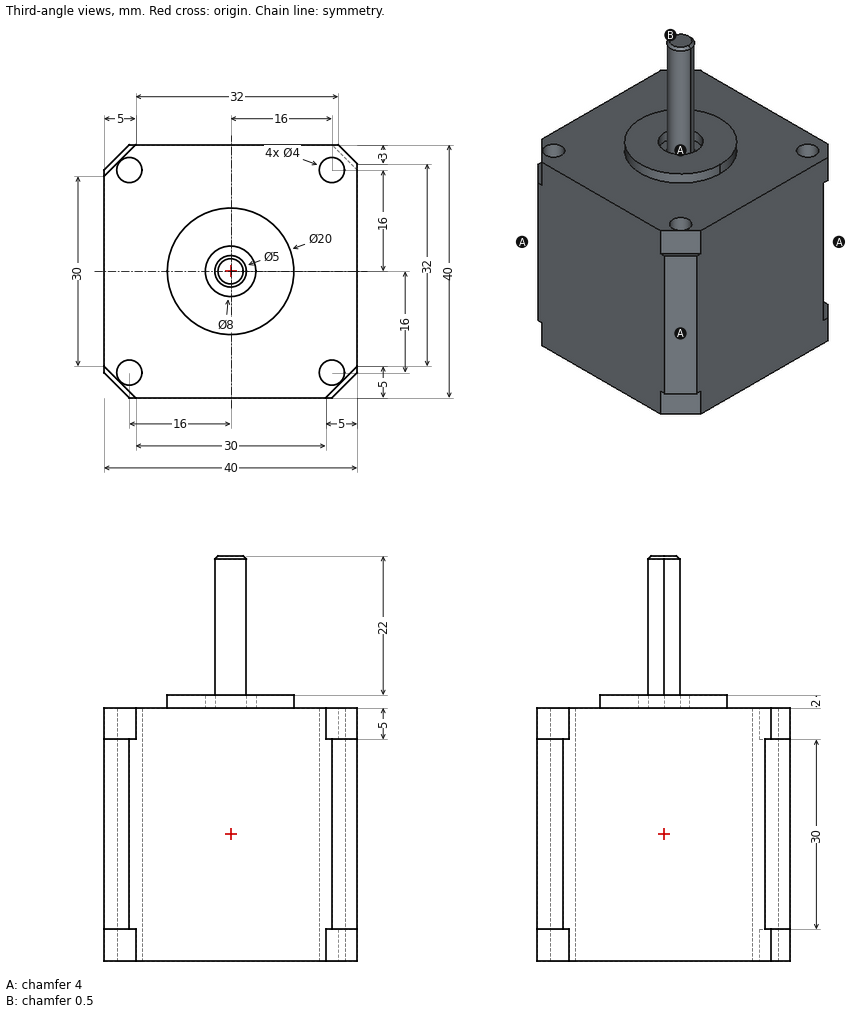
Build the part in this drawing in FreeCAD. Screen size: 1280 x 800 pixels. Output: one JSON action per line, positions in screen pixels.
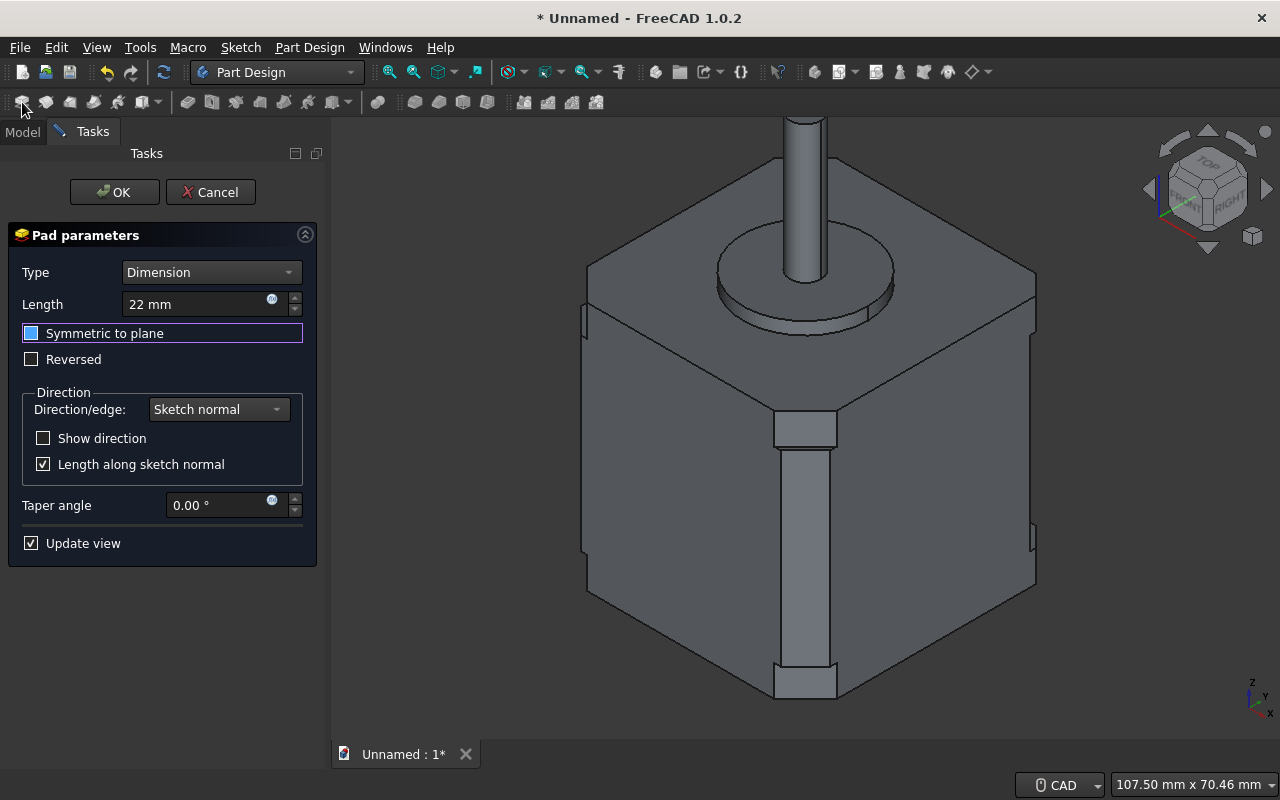
{"action": "left_click", "coordinate": [115, 192]}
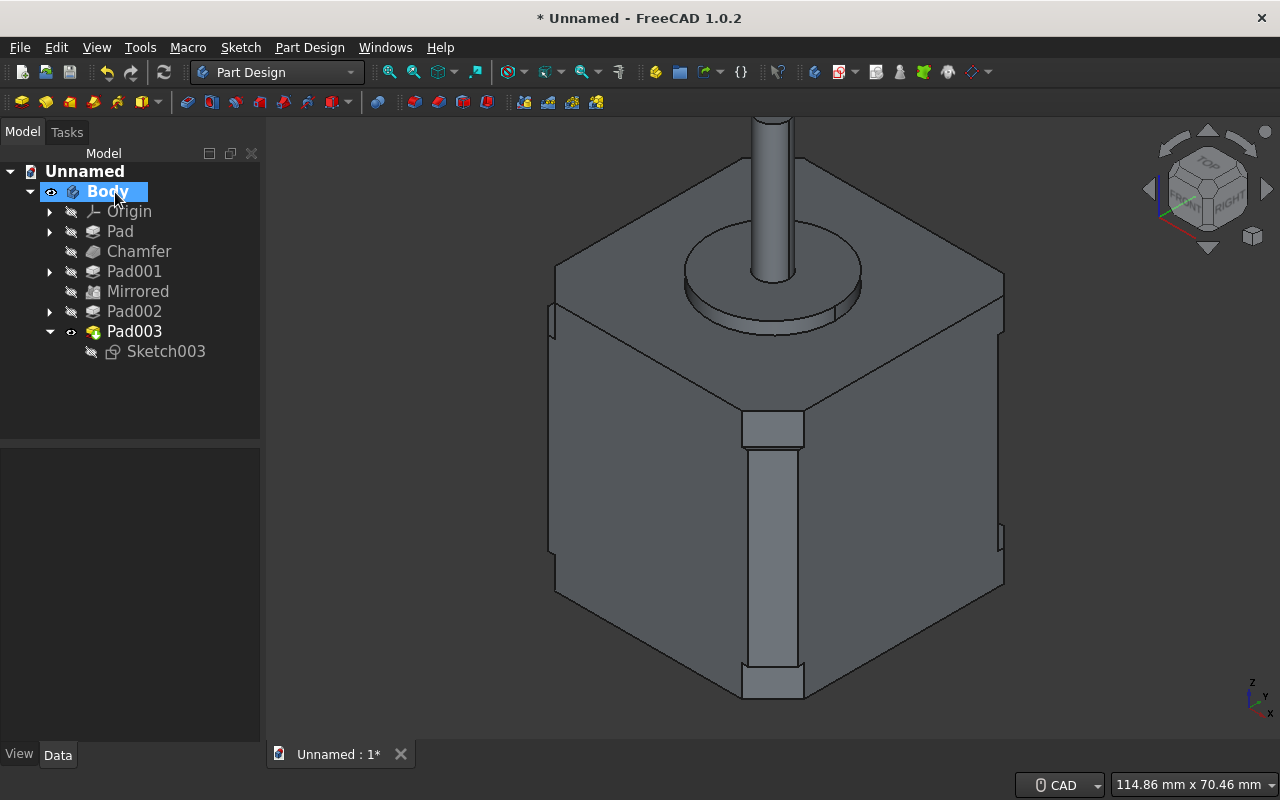
{"action": "left_click", "coordinate": [390, 72]}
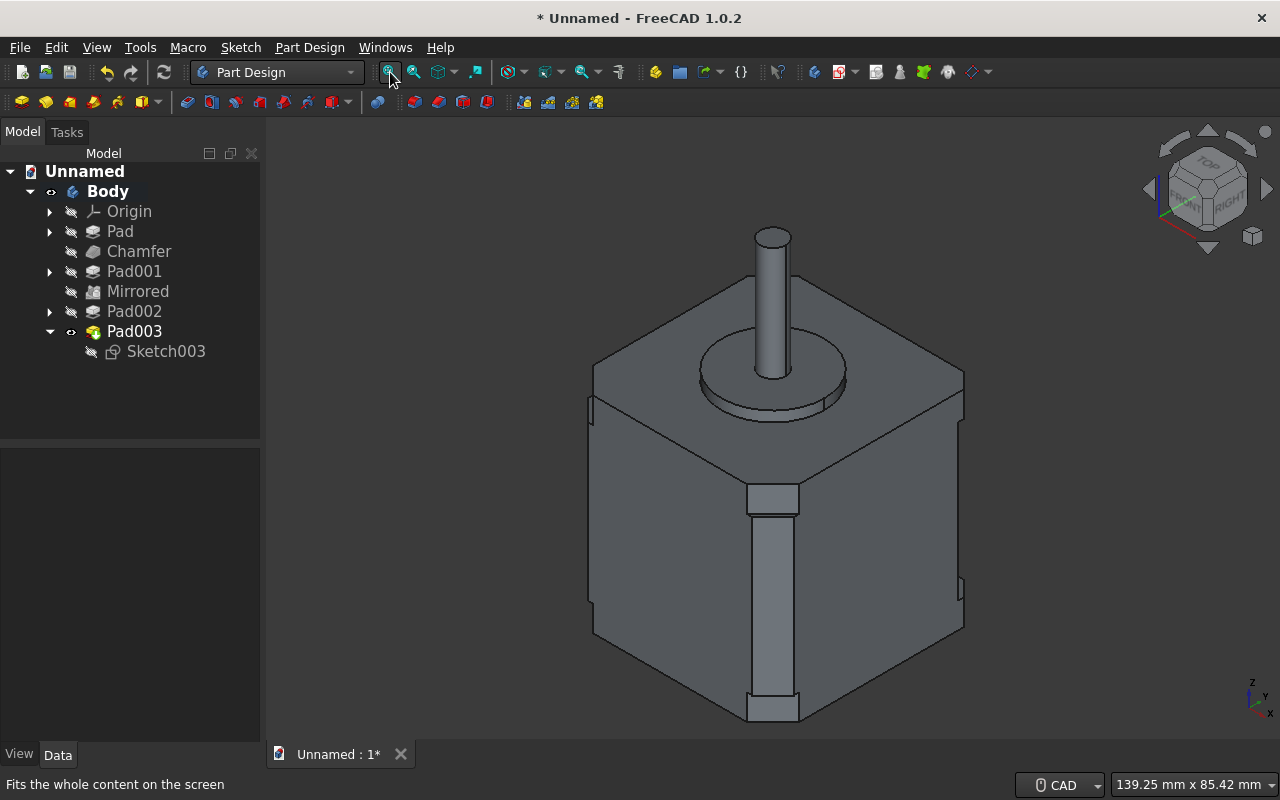
{"action": "left_click", "coordinate": [655, 379]}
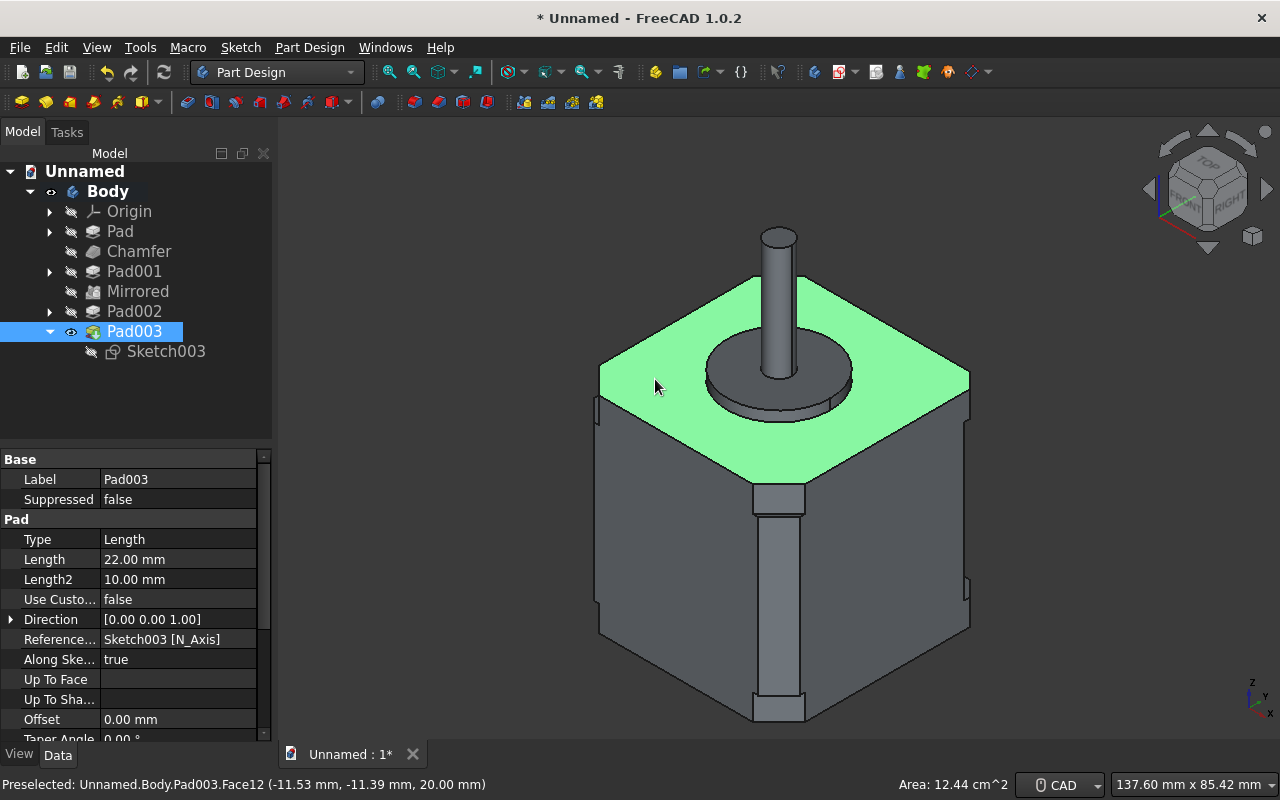
{"action": "left_click", "coordinate": [840, 72]}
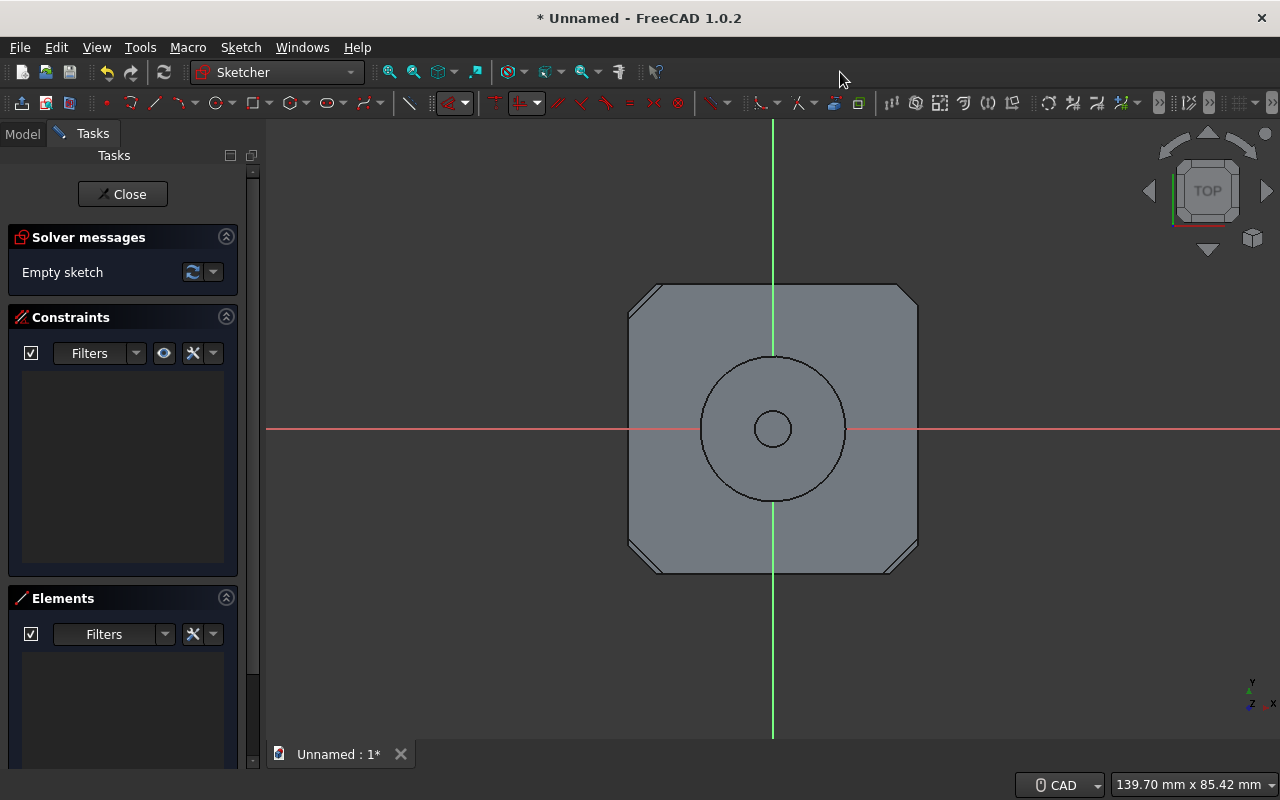
{"action": "left_click", "coordinate": [70, 104]}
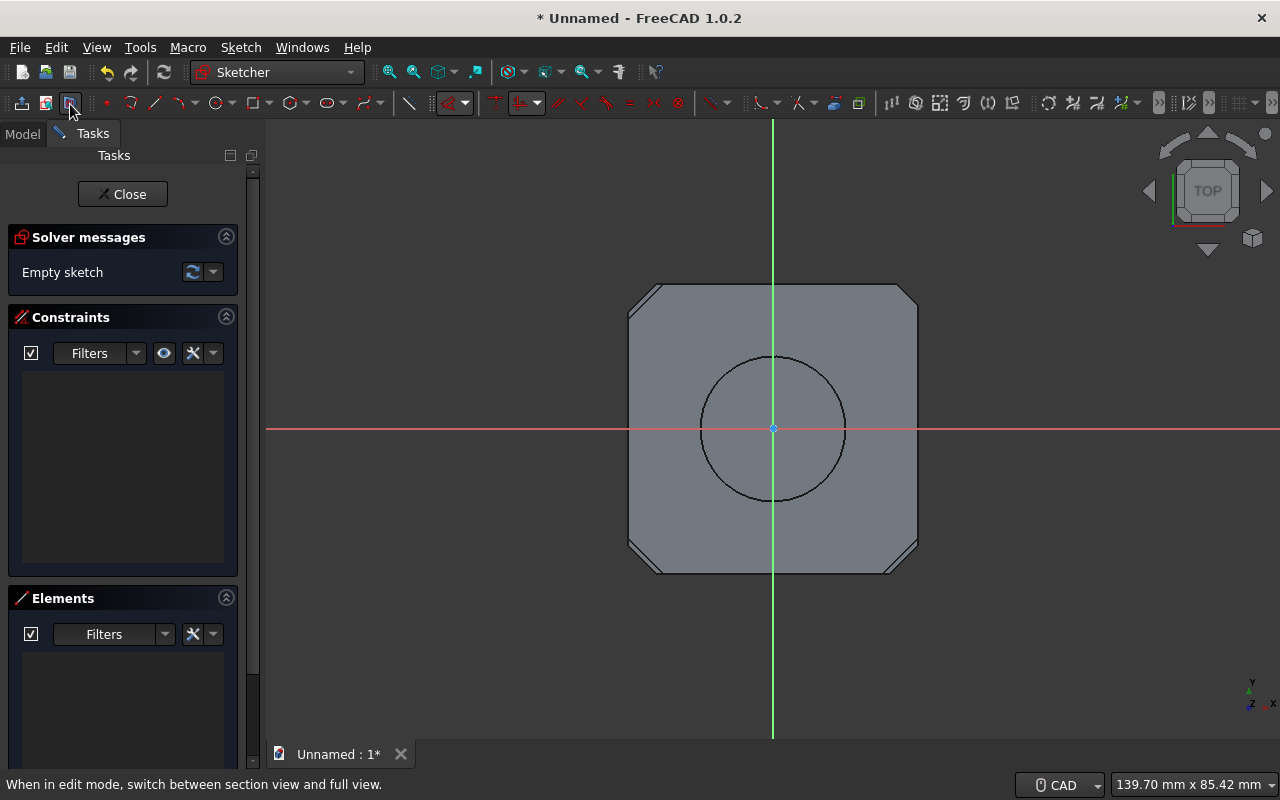
{"action": "scroll", "coordinate": [784, 429], "scroll_direction": "up", "scroll_amount": 10}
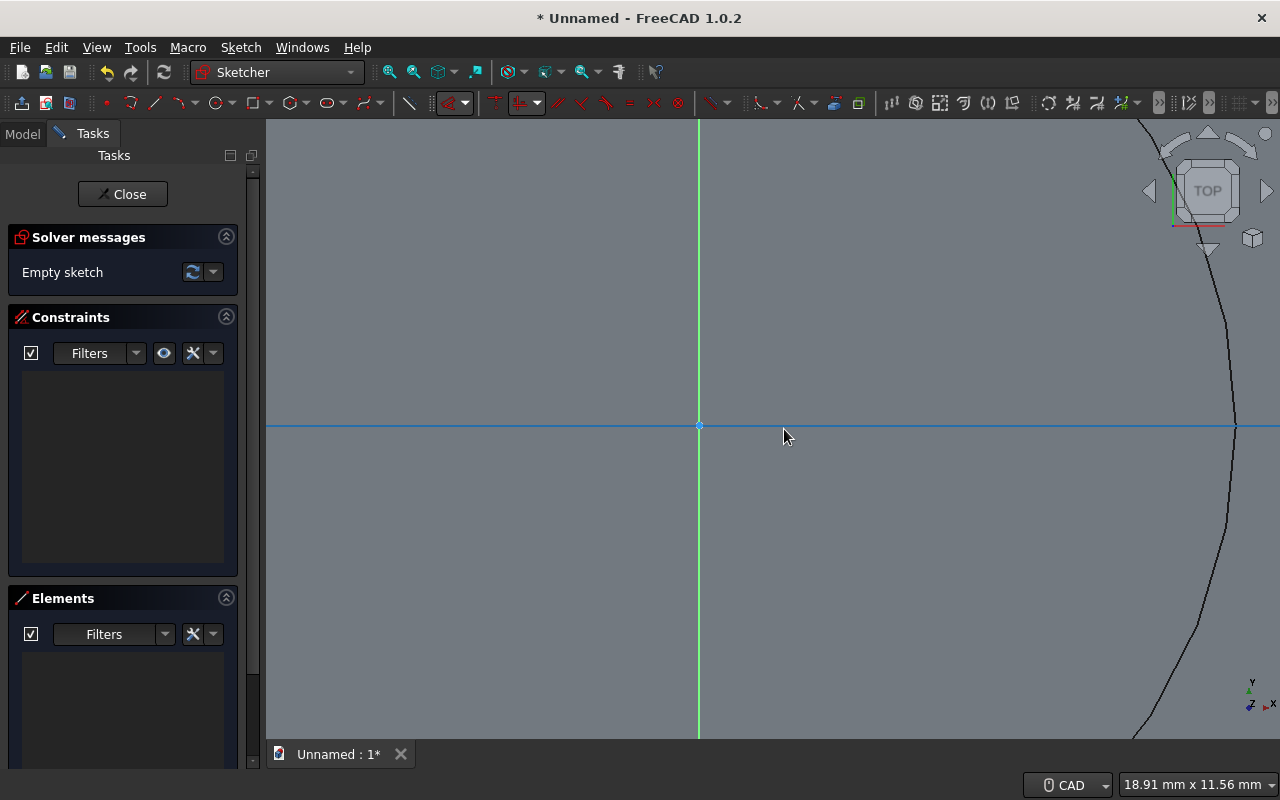
{"action": "left_click", "coordinate": [216, 104]}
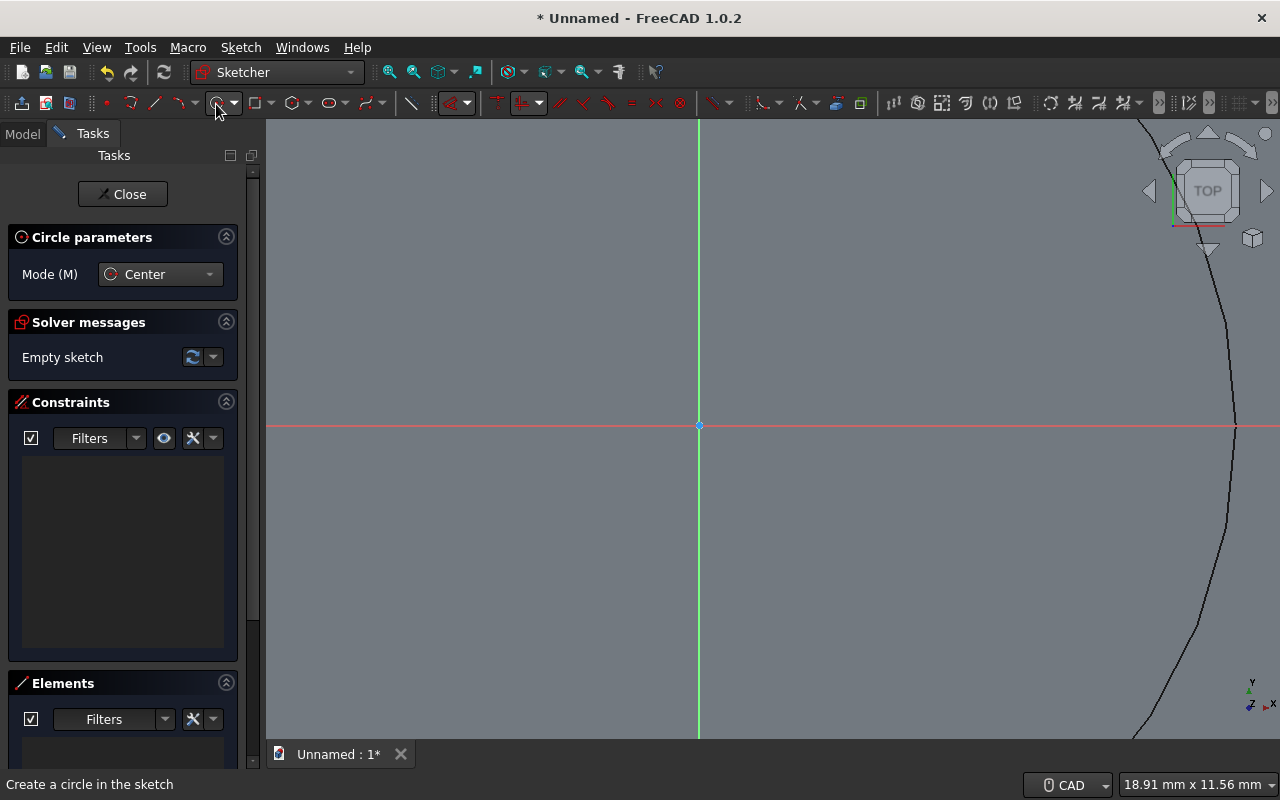
{"action": "left_click", "coordinate": [699, 426]}
{"action": "mouse_move", "coordinate": [851, 274]}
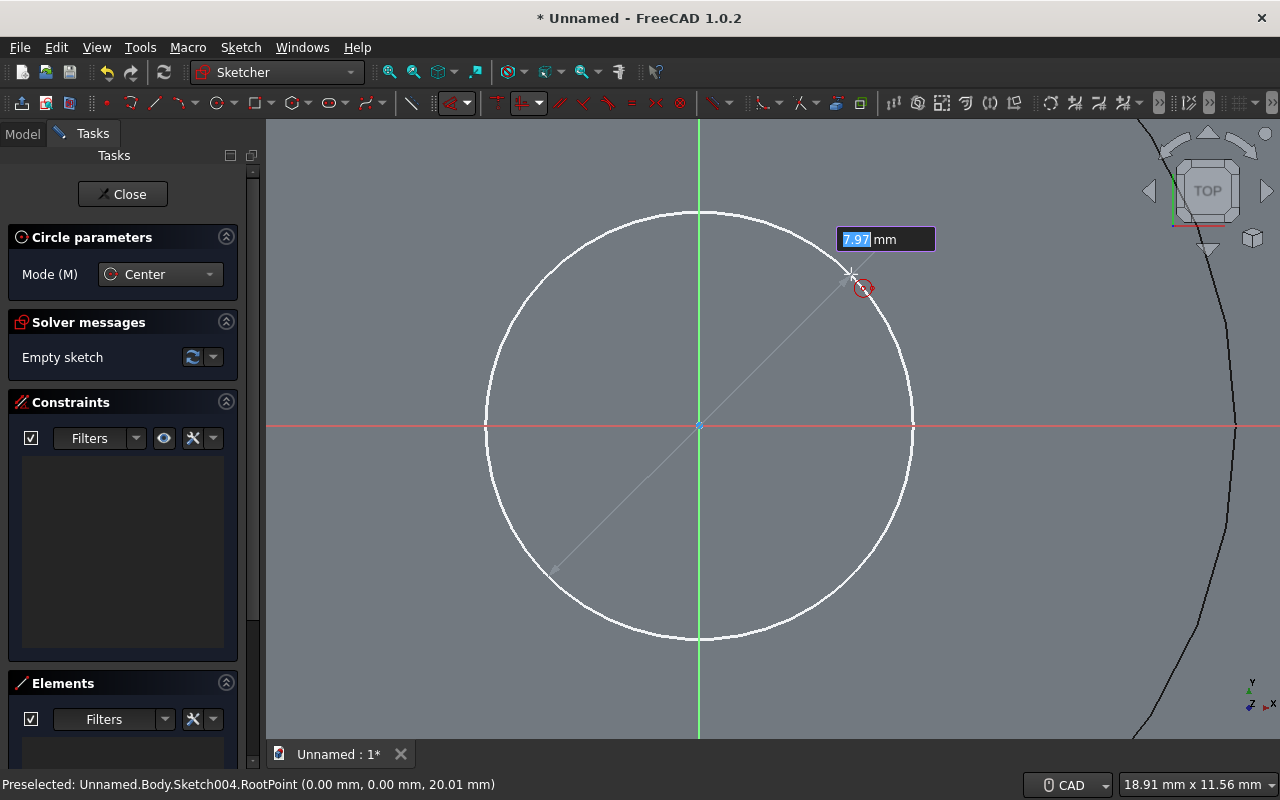
{"action": "type", "text": "8"}
{"action": "key", "text": "Return"}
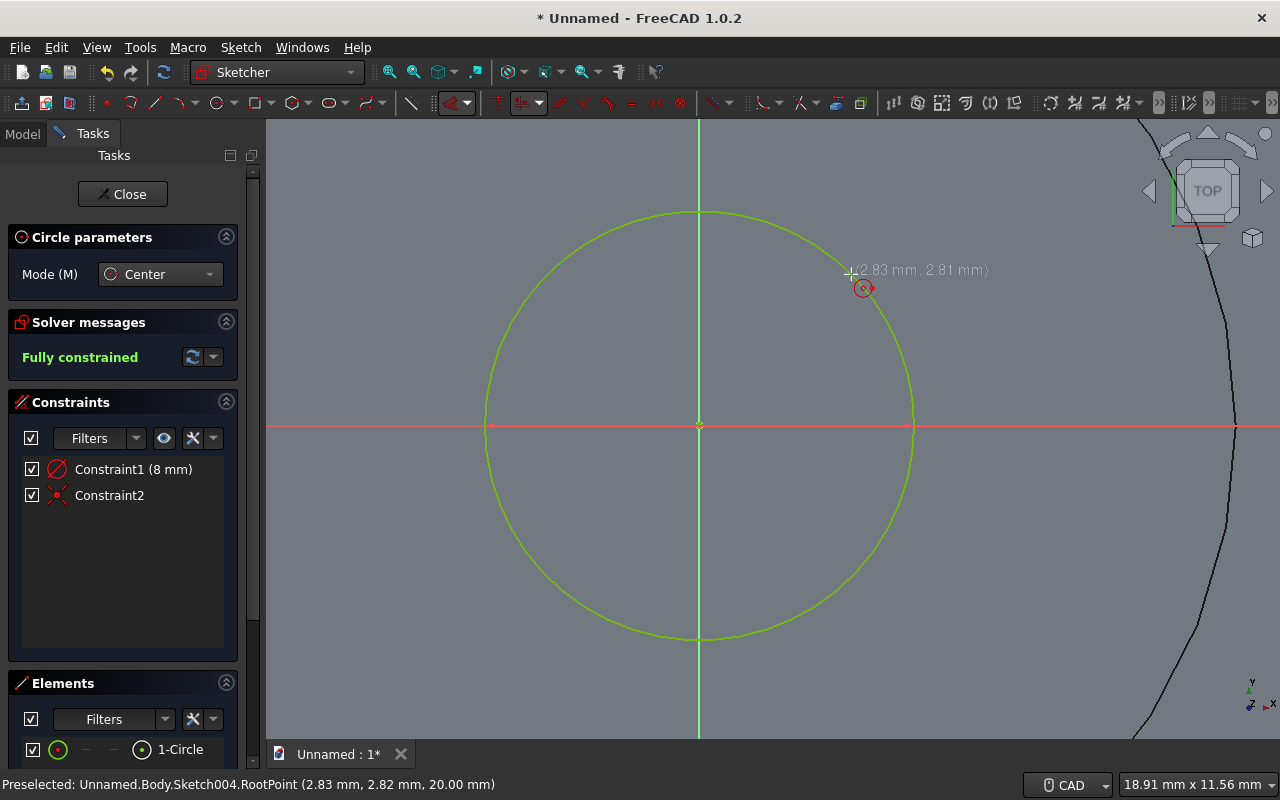
{"action": "left_click", "coordinate": [699, 426]}
{"action": "mouse_move", "coordinate": [794, 331]}